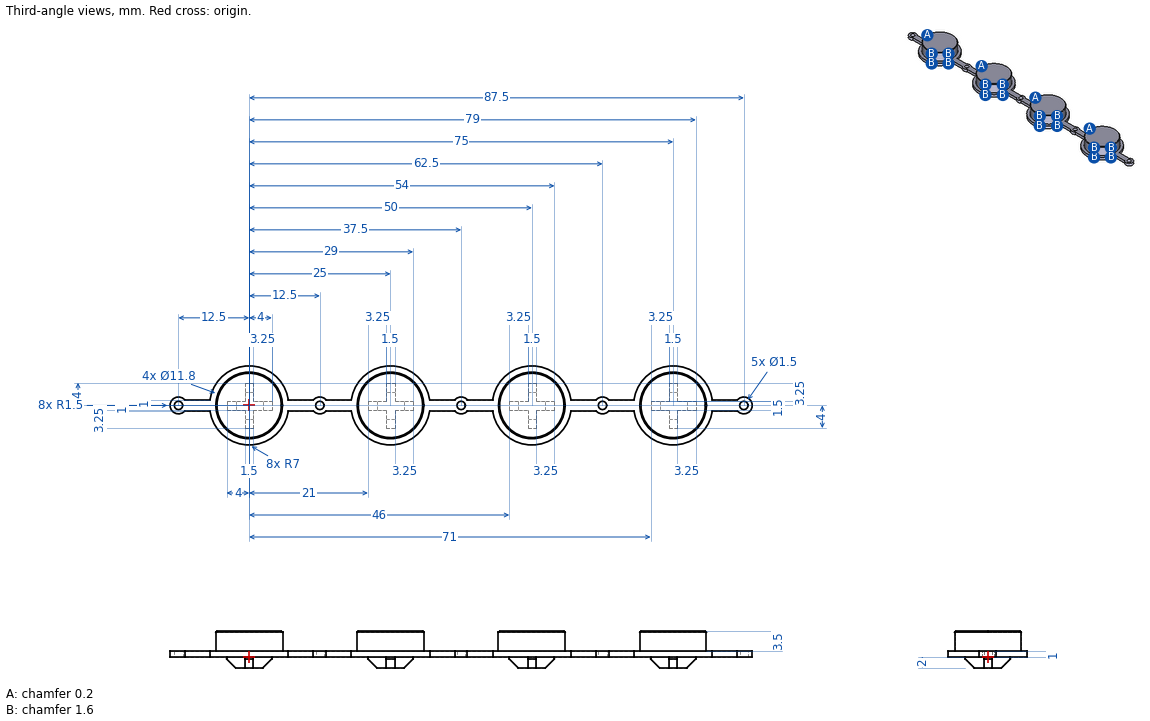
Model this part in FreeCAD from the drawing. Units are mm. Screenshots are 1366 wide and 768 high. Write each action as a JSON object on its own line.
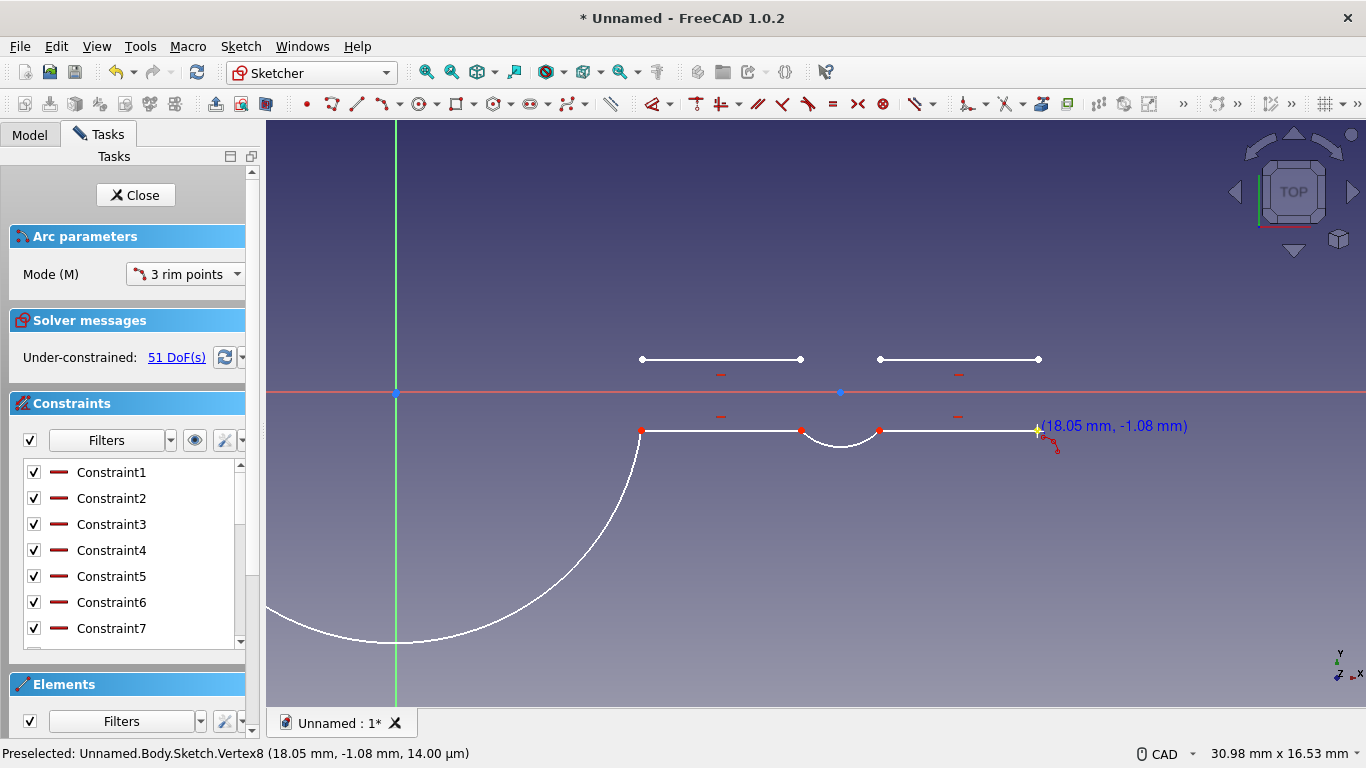
{"action": "scroll", "coordinate": [553, 418], "scroll_direction": "down", "scroll_amount": 9}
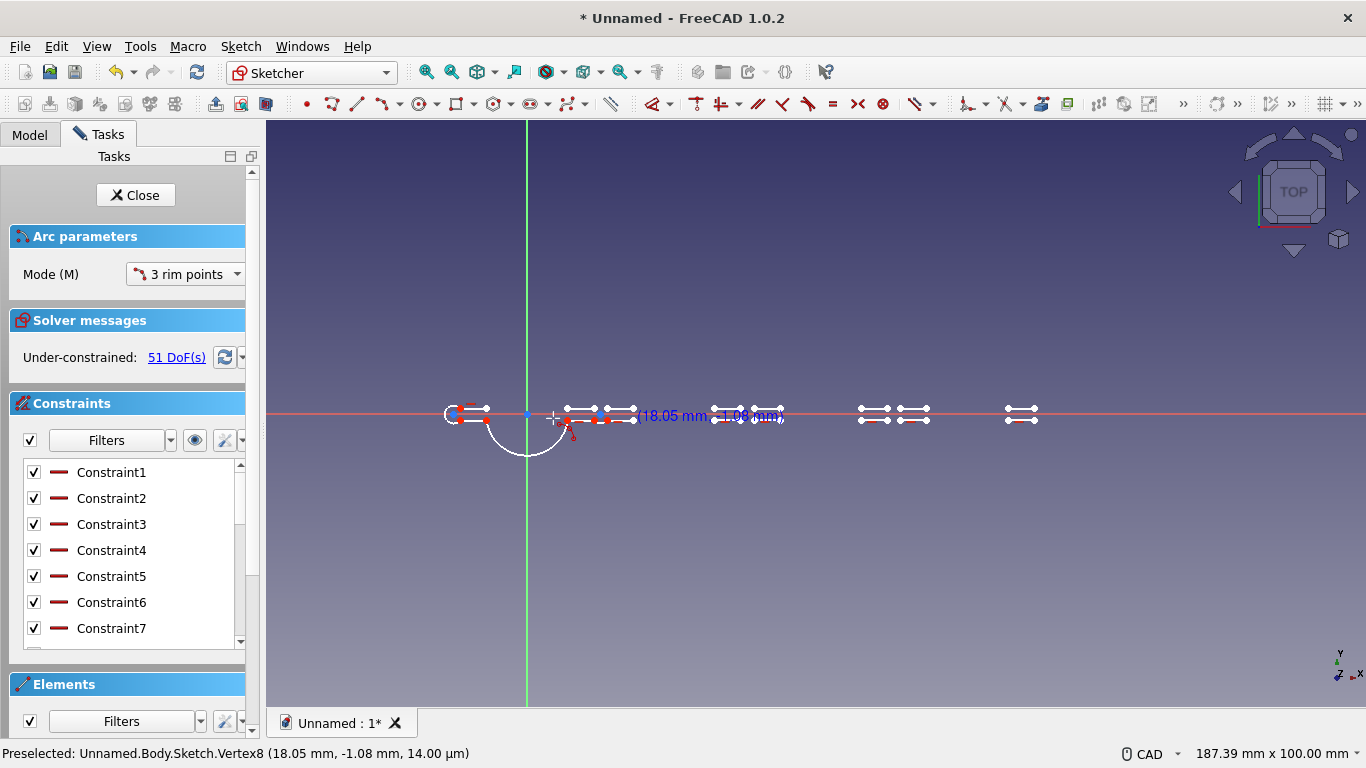
{"action": "scroll", "coordinate": [715, 420], "scroll_direction": "up", "scroll_amount": 5}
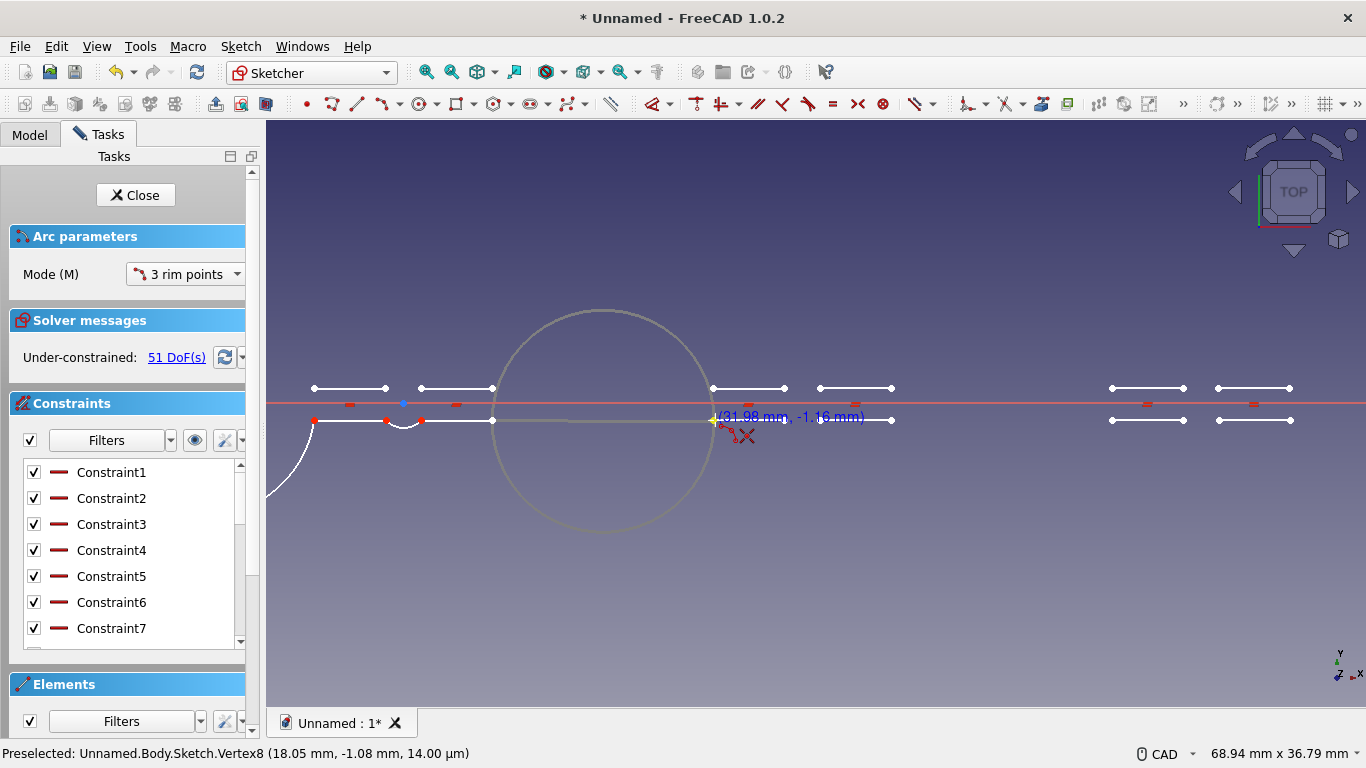
{"action": "left_click", "coordinate": [713, 420]}
{"action": "left_click", "coordinate": [603, 515]}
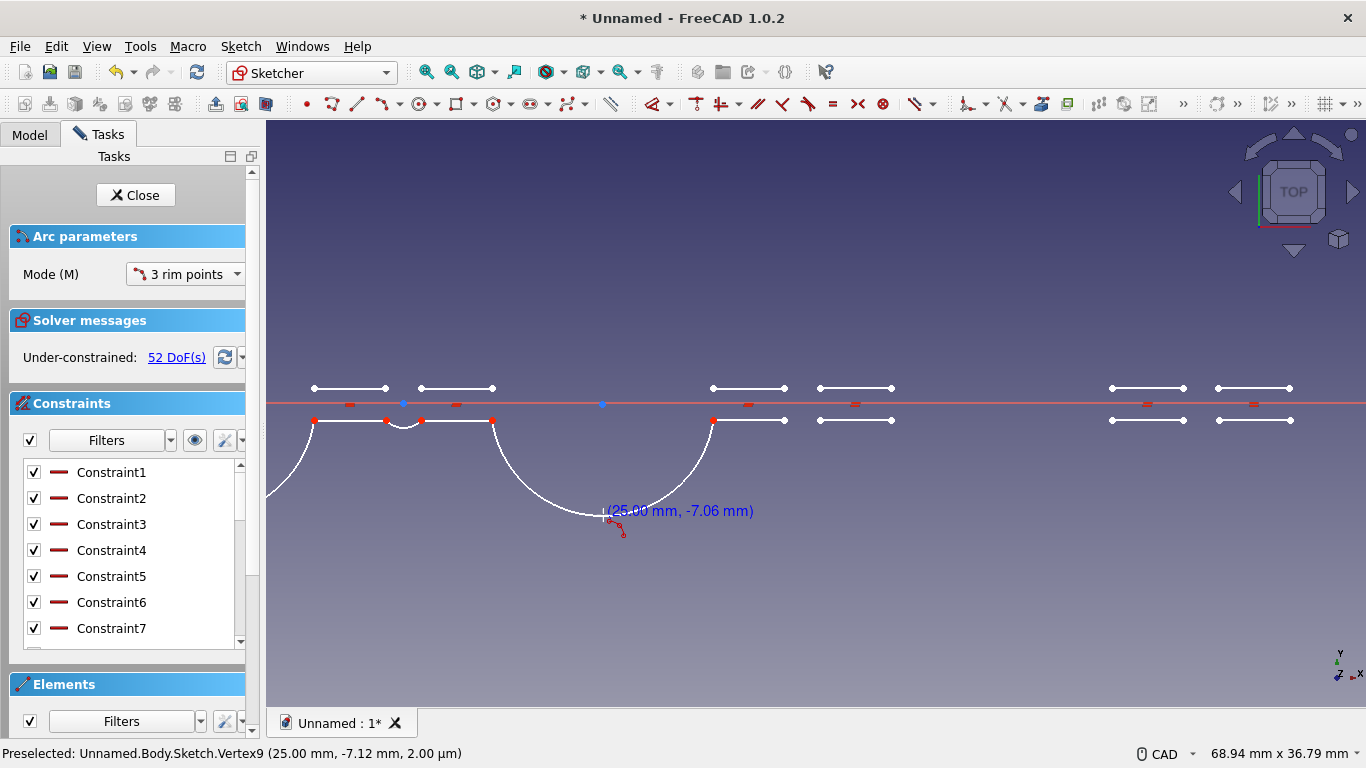
{"action": "left_click", "coordinate": [784, 420]}
{"action": "left_click", "coordinate": [820, 420]}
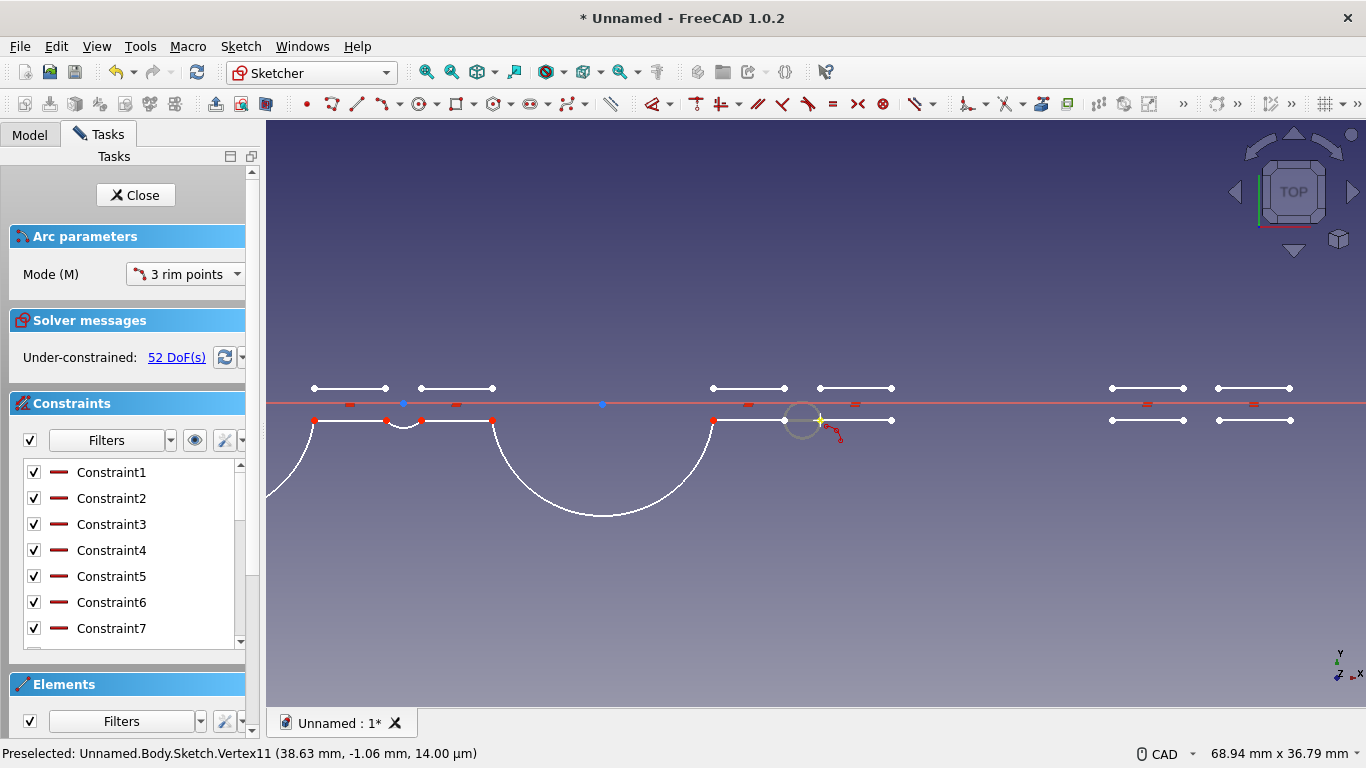
{"action": "scroll", "coordinate": [802, 427], "scroll_direction": "up", "scroll_amount": 4}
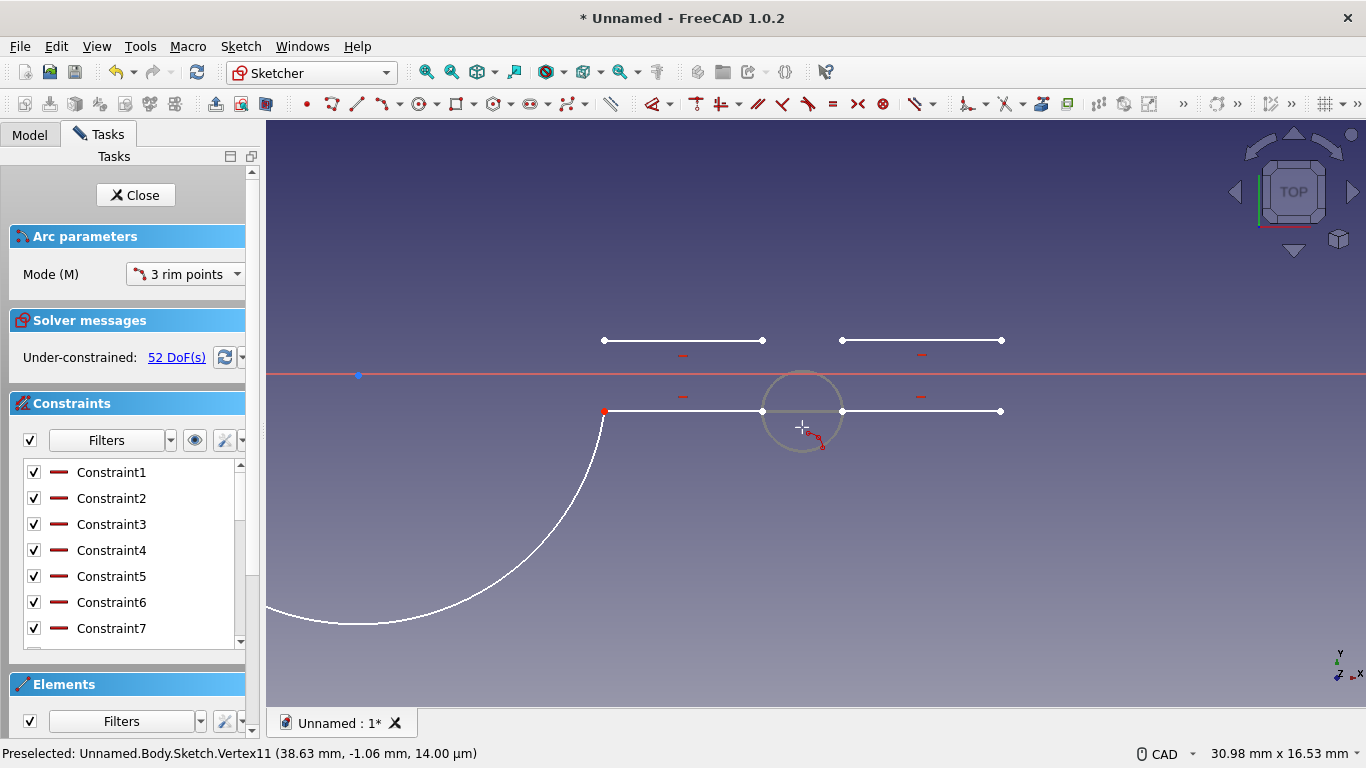
{"action": "left_click", "coordinate": [802, 427]}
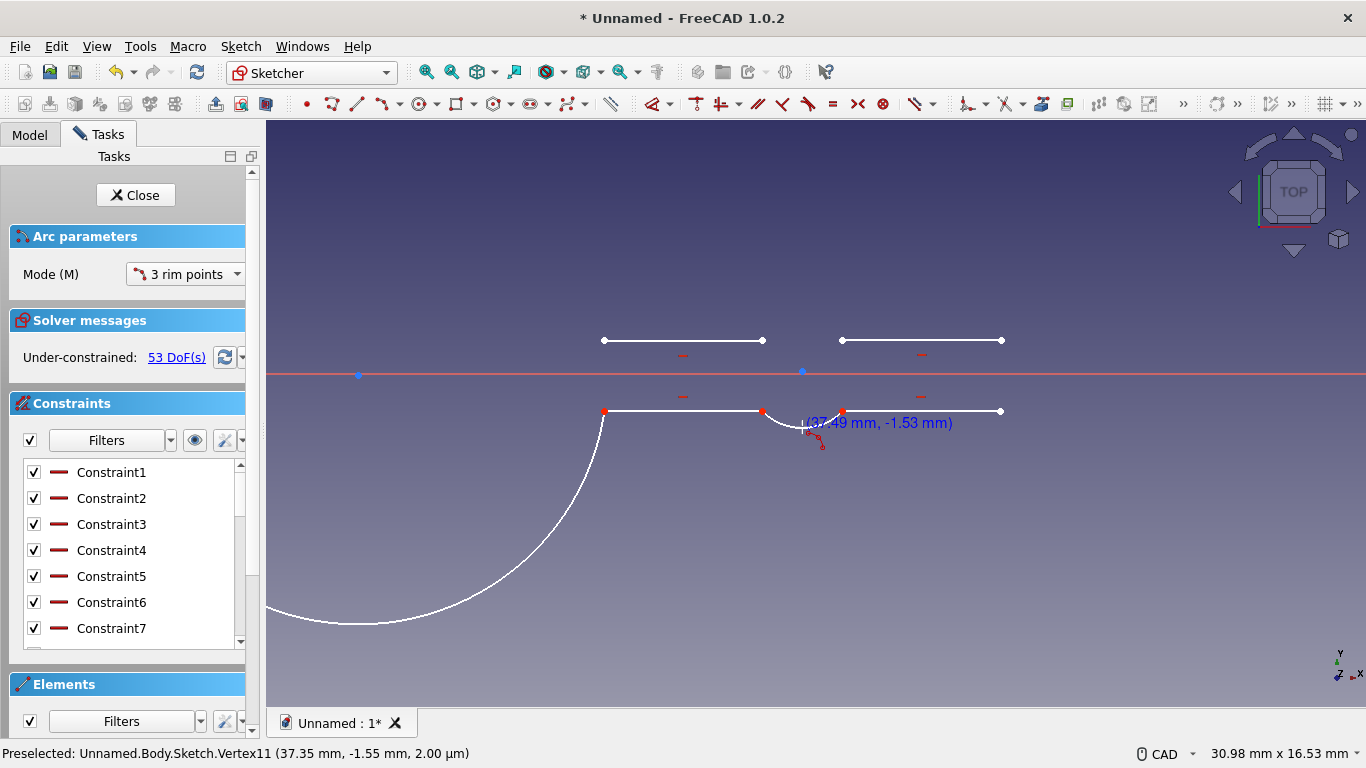
{"action": "left_click", "coordinate": [1001, 411]}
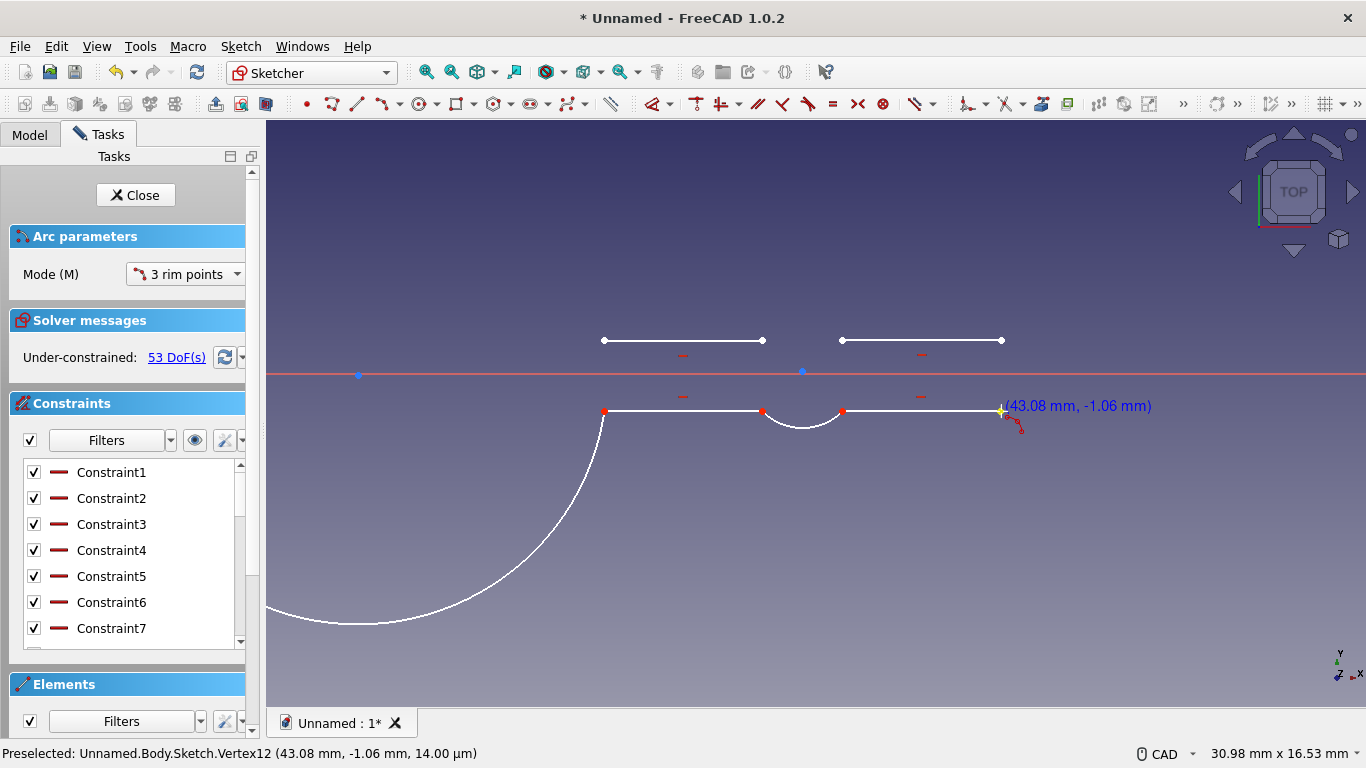
{"action": "scroll", "coordinate": [737, 421], "scroll_direction": "down", "scroll_amount": 9}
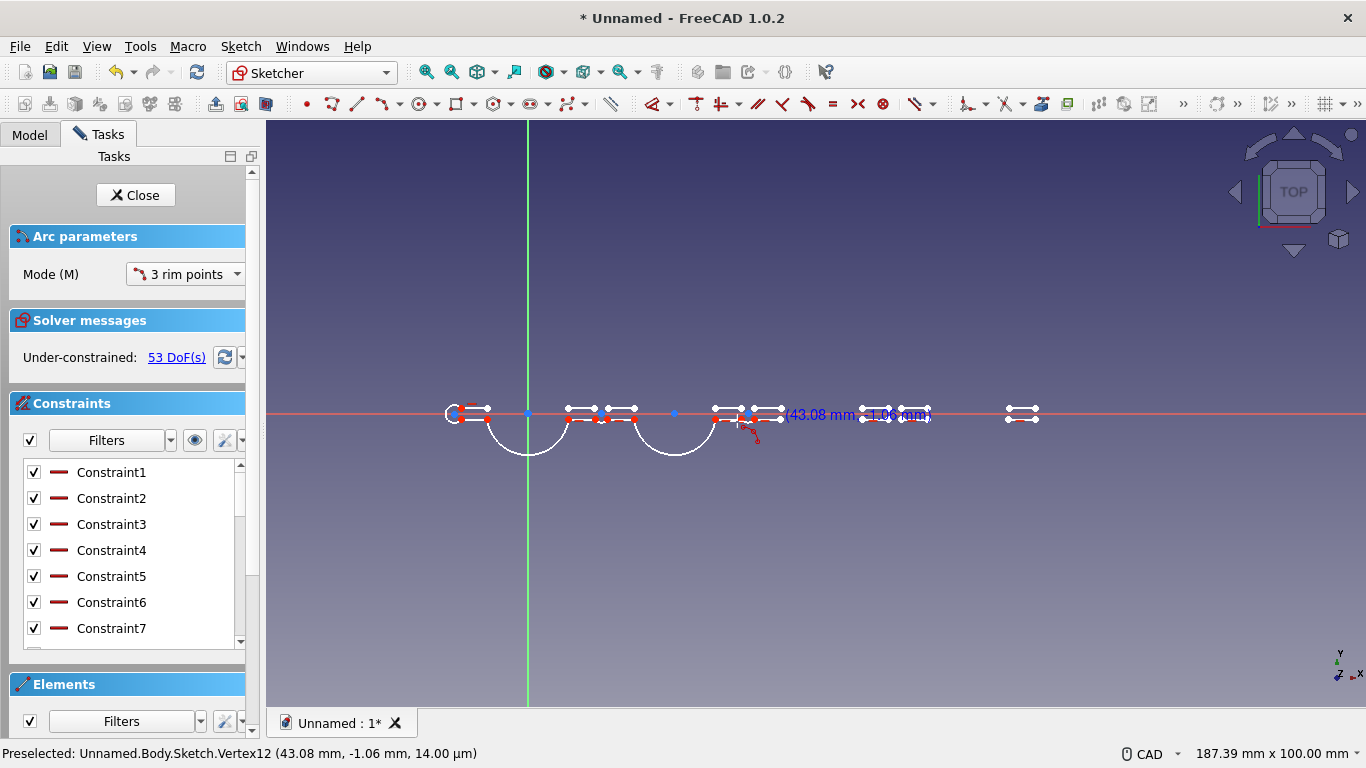
{"action": "scroll", "coordinate": [862, 419], "scroll_direction": "up", "scroll_amount": 5}